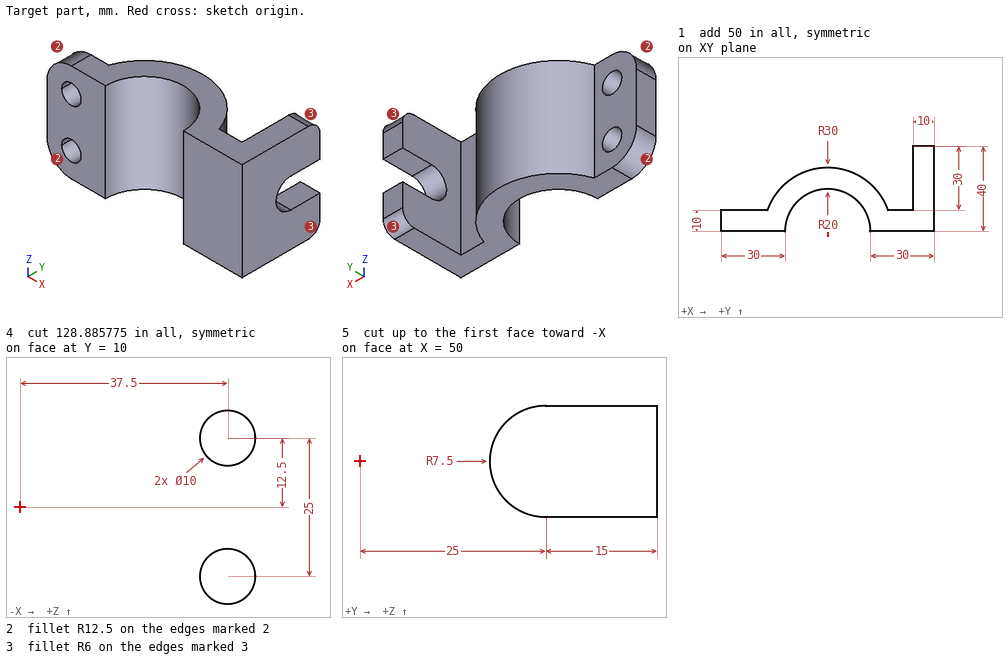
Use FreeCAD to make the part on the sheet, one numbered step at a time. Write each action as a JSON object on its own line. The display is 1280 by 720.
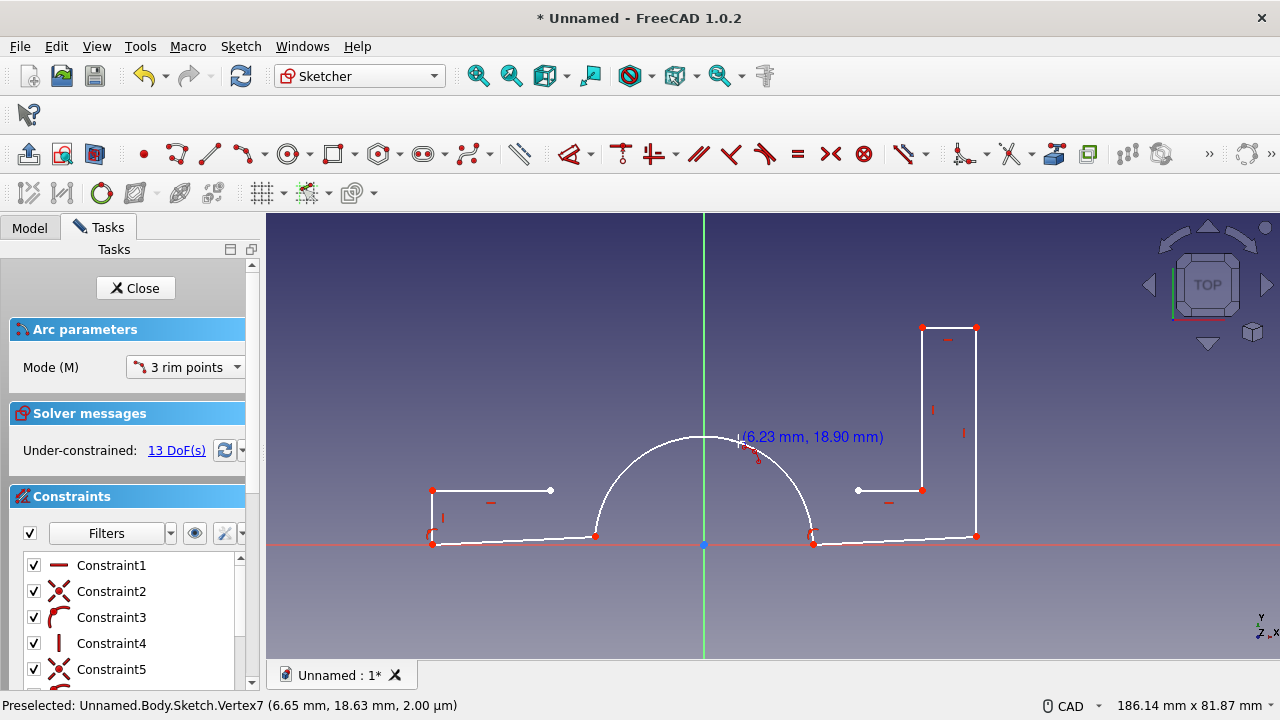
{"action": "left_click", "coordinate": [858, 491]}
{"action": "left_click", "coordinate": [550, 491]}
{"action": "left_click", "coordinate": [744, 386]}
{"action": "key", "text": "Escape"}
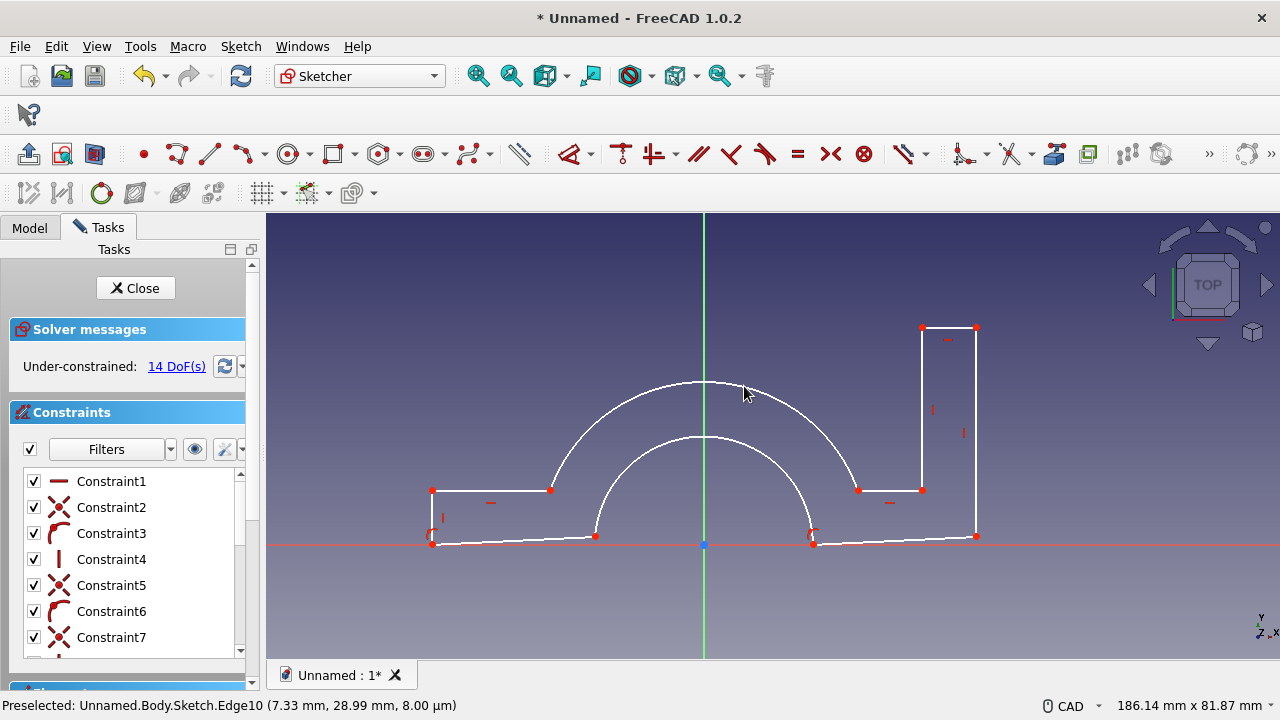
{"action": "left_click", "coordinate": [481, 543]}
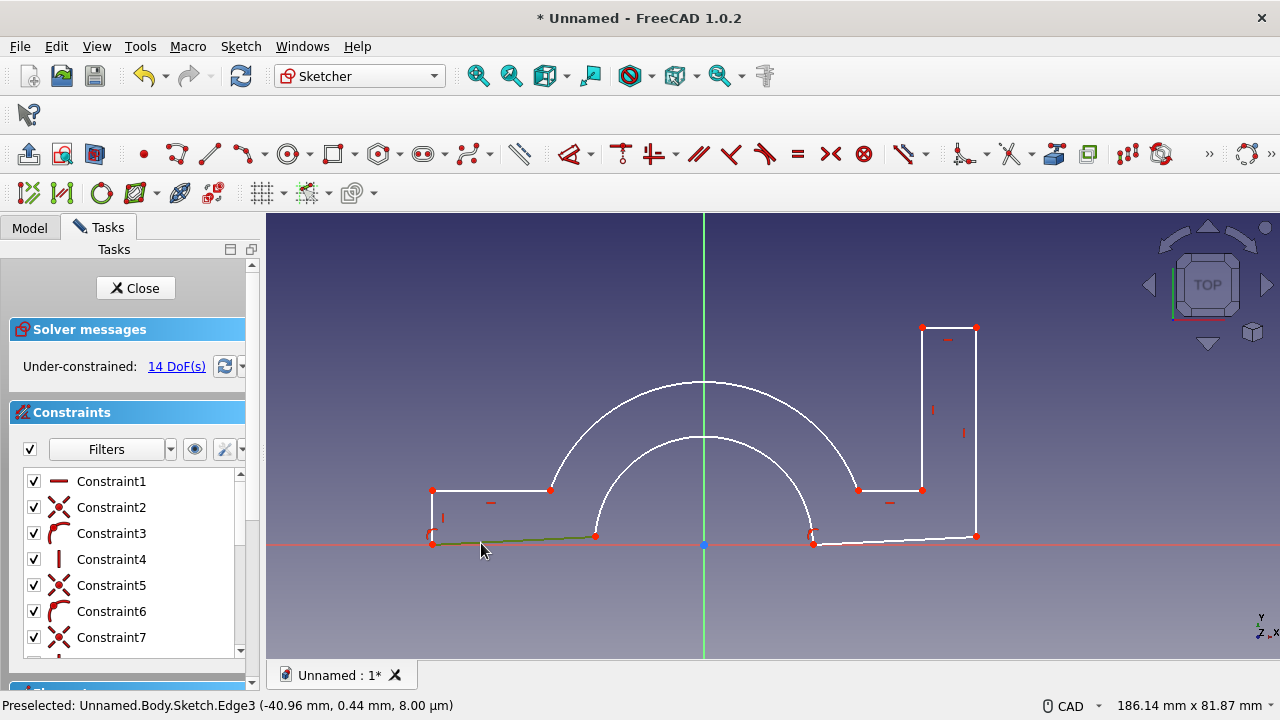
{"action": "left_click", "coordinate": [676, 154]}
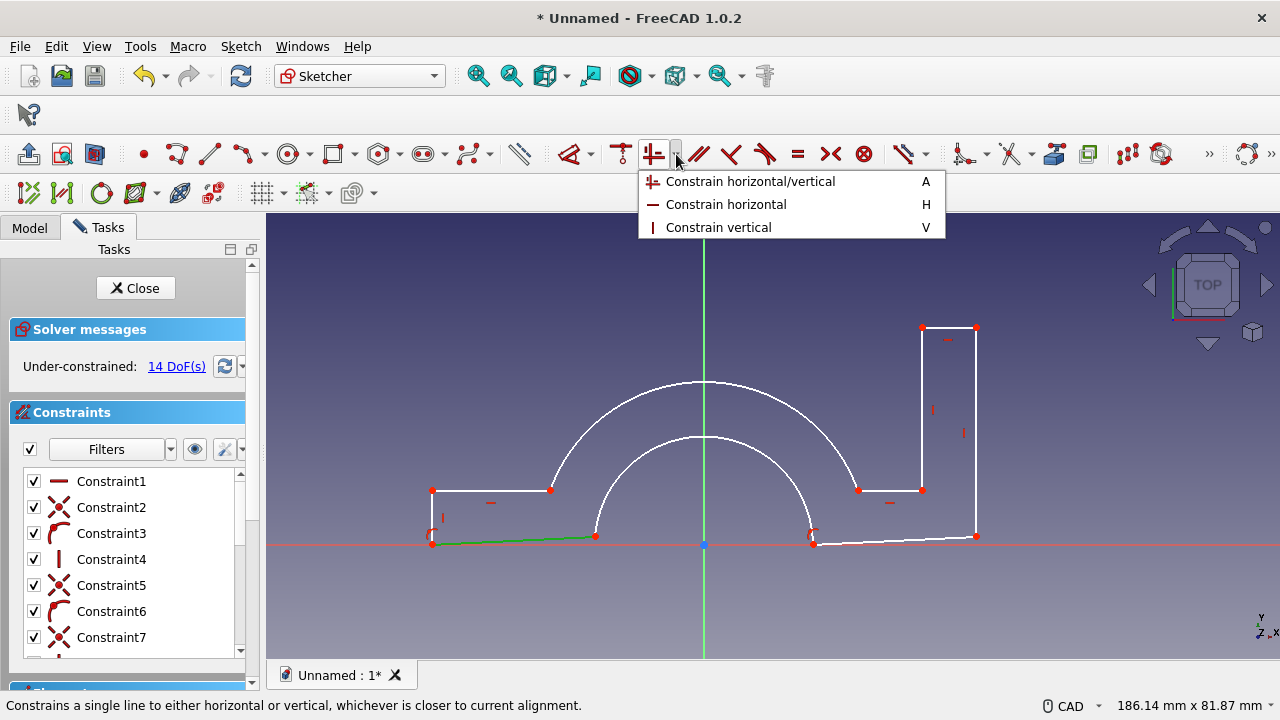
{"action": "left_click", "coordinate": [792, 204]}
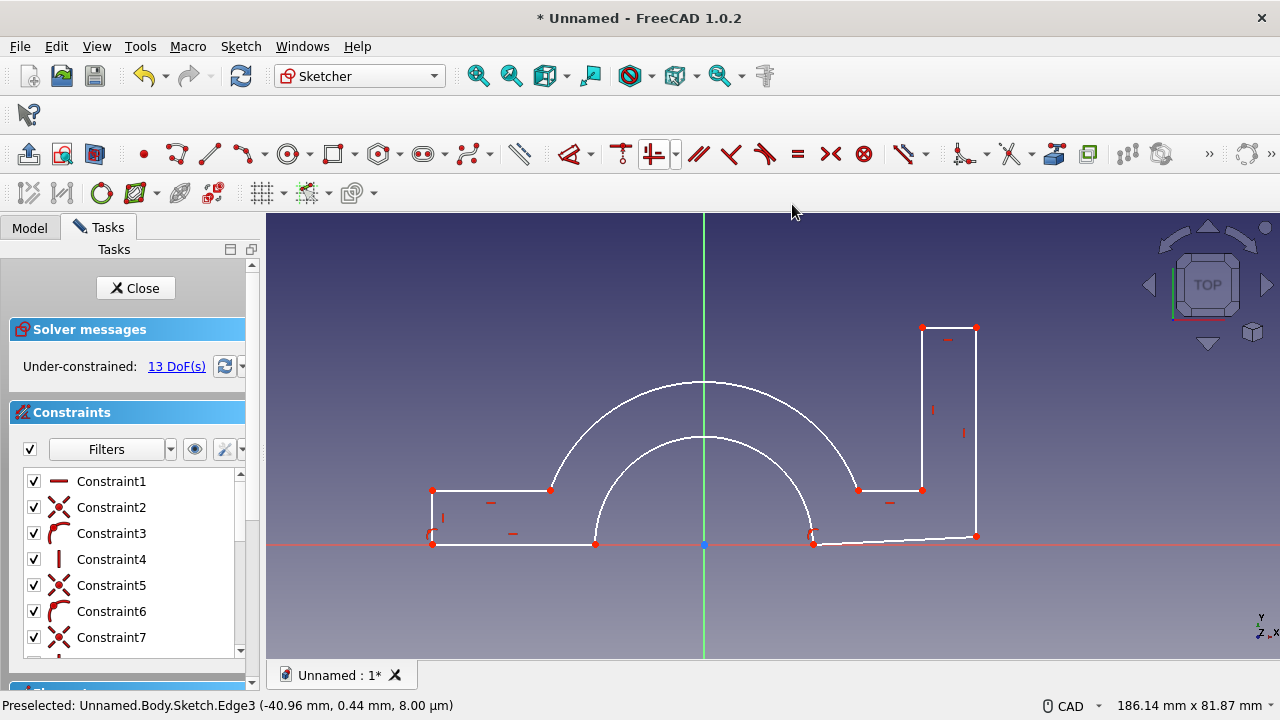
{"action": "left_click", "coordinate": [862, 543]}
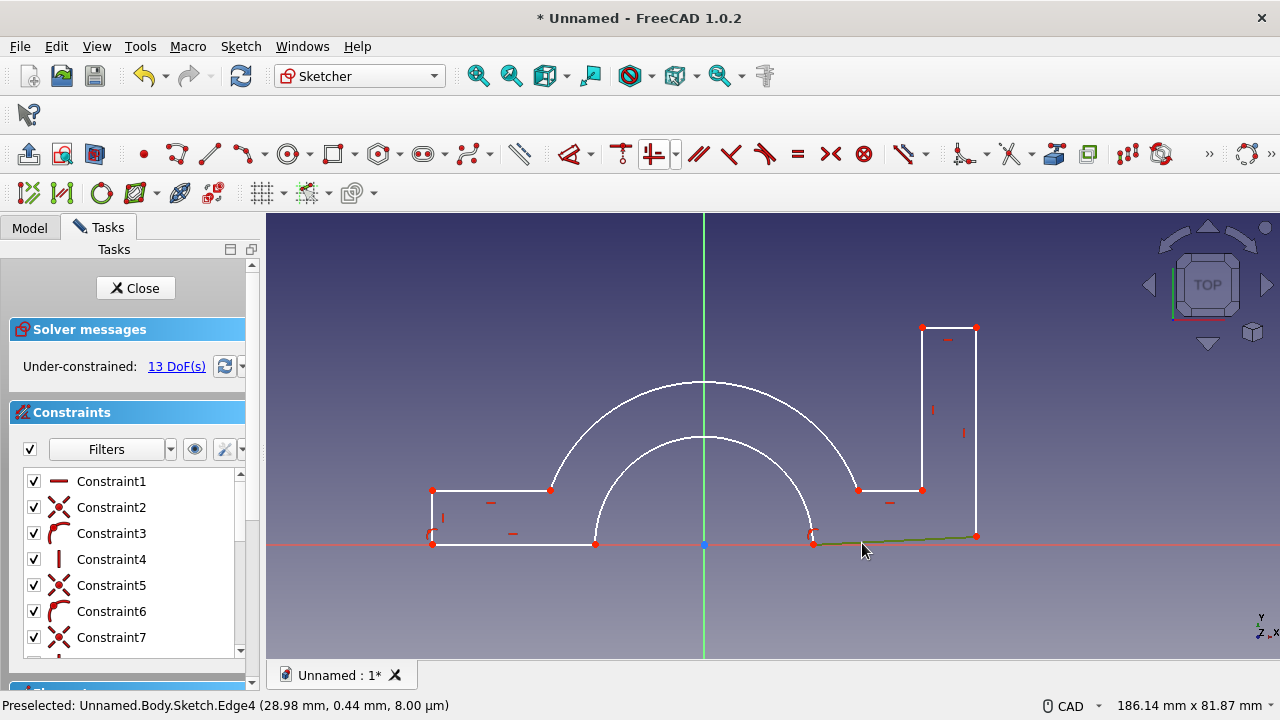
{"action": "key", "text": "h"}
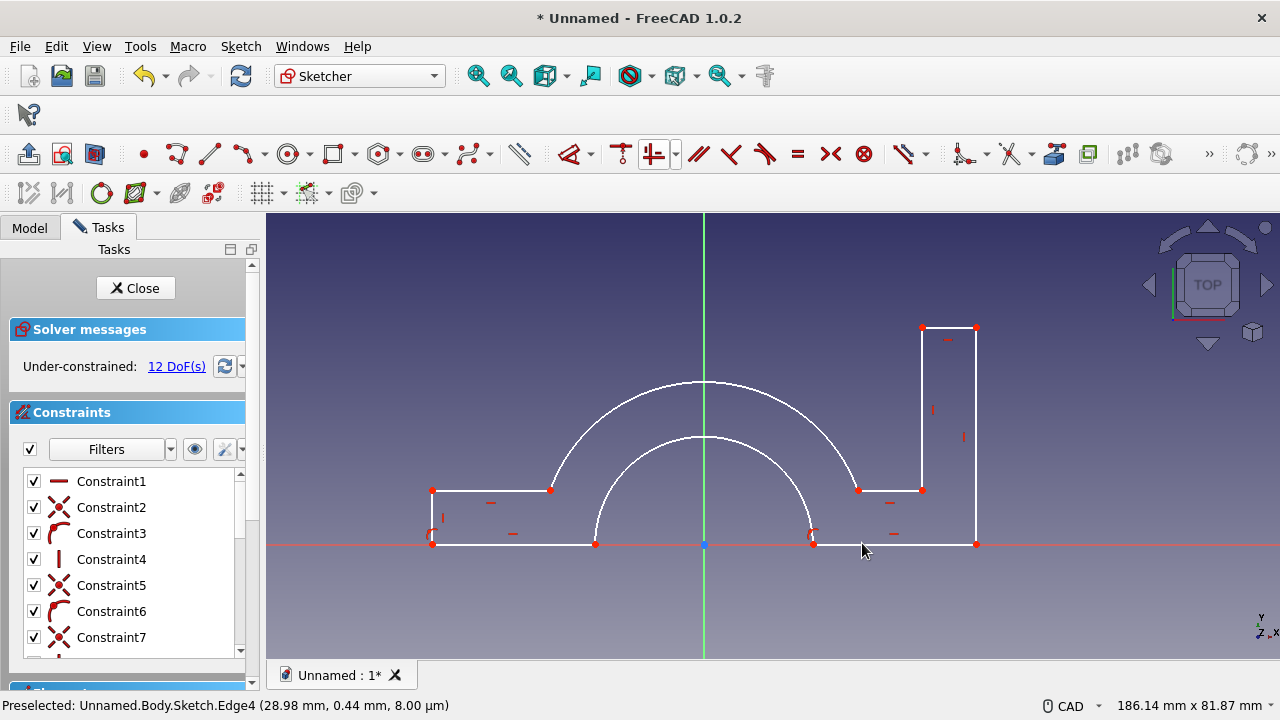
{"action": "left_click", "coordinate": [768, 457]}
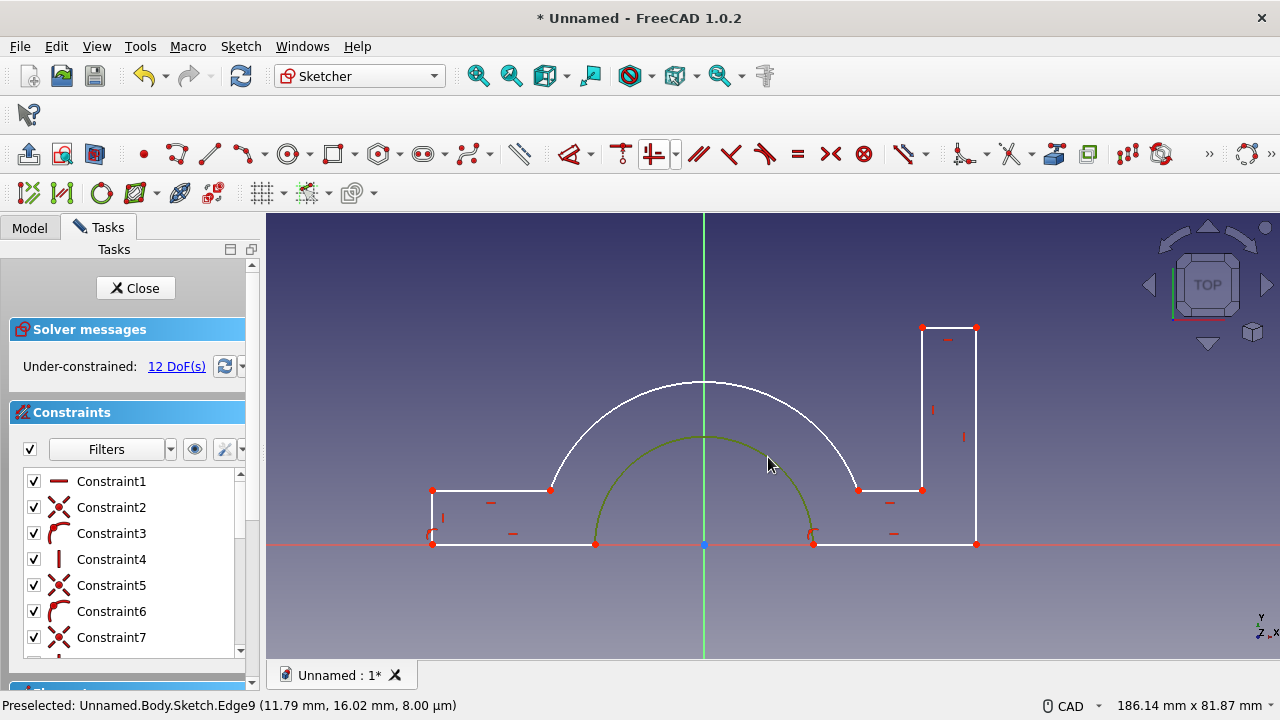
{"action": "left_click", "coordinate": [781, 401]}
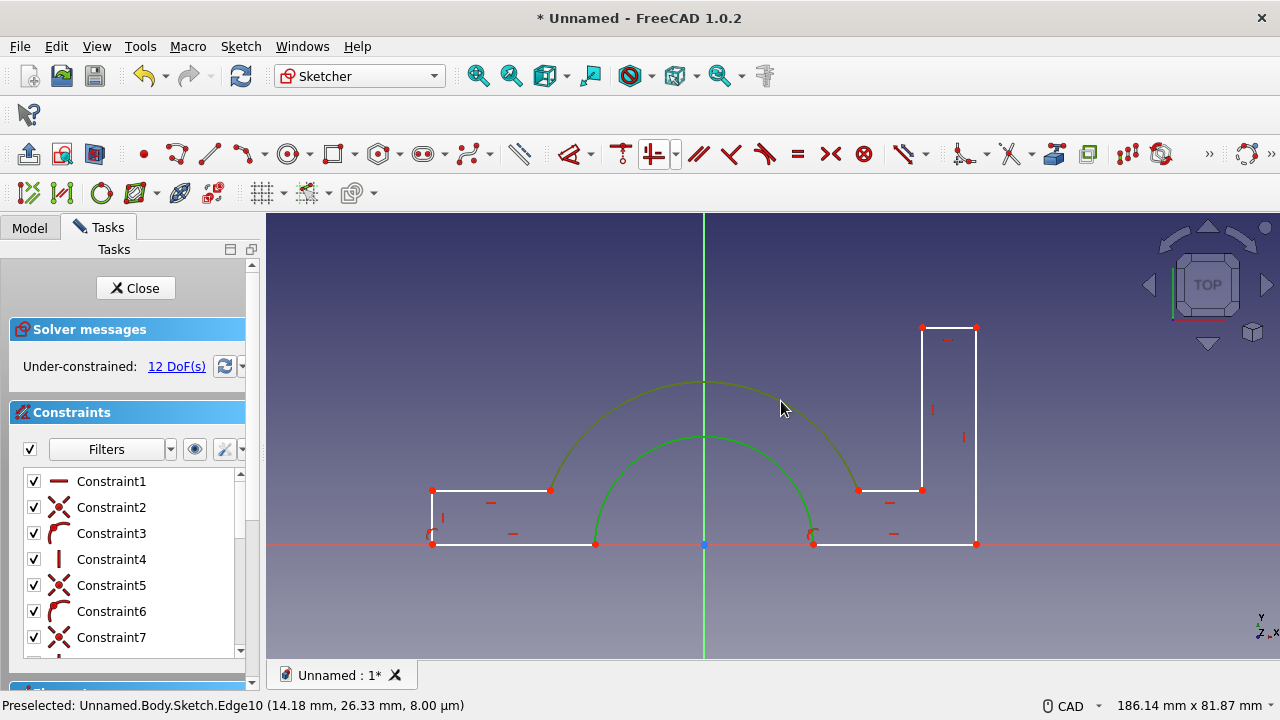
{"action": "left_click", "coordinate": [621, 154]}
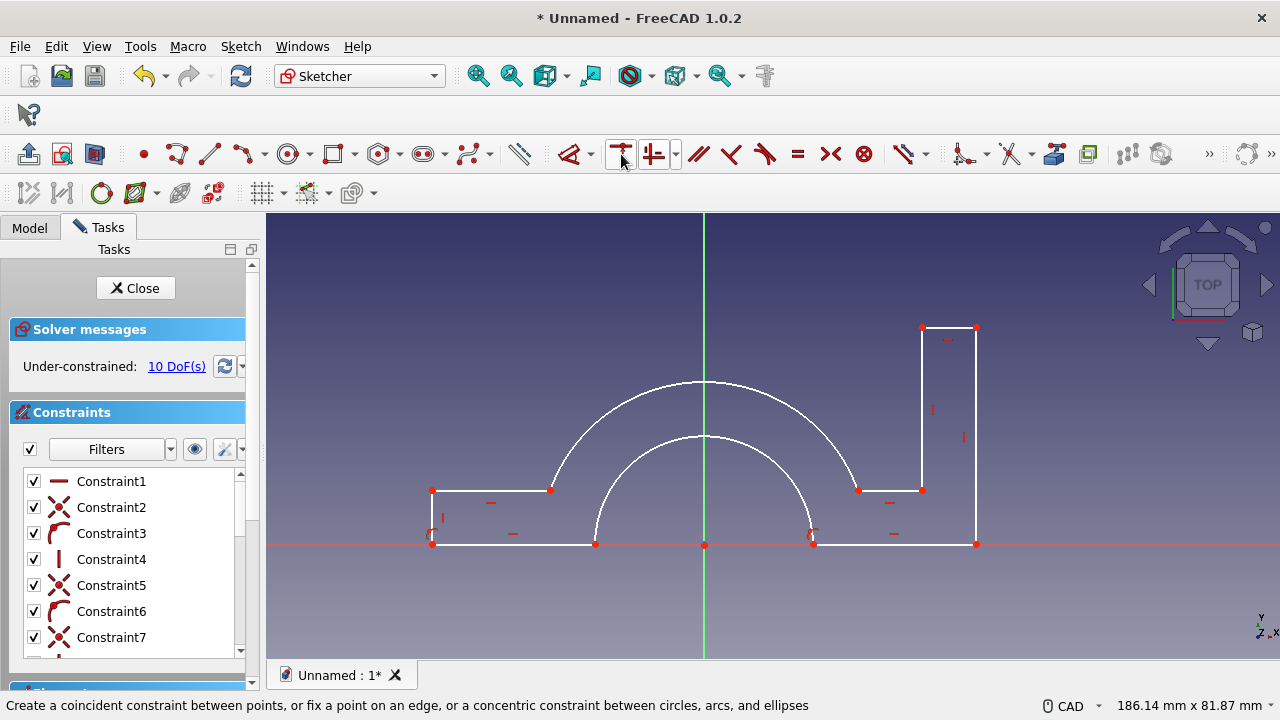
{"action": "left_click_drag", "start_coordinate": [694, 535], "coordinate": [714, 555]}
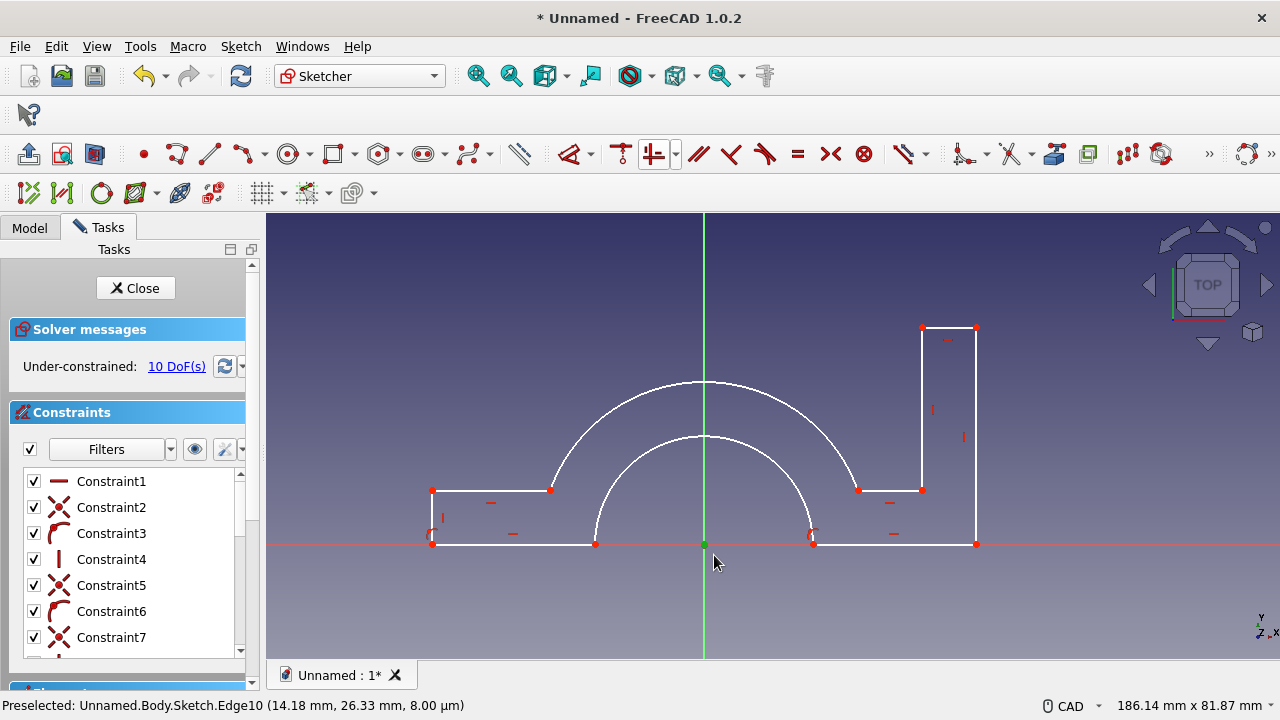
{"action": "left_click", "coordinate": [621, 154]}